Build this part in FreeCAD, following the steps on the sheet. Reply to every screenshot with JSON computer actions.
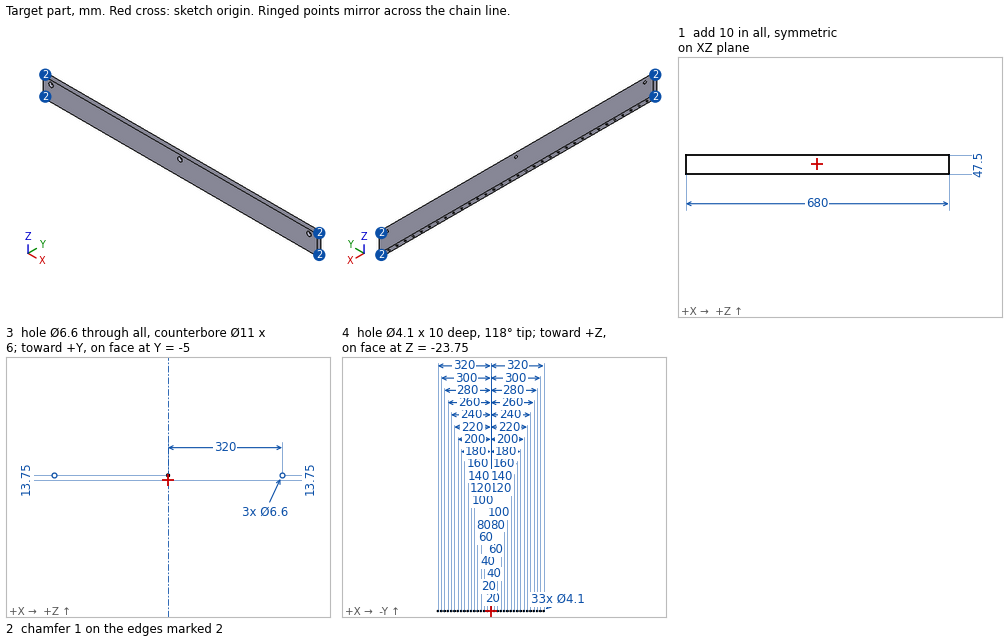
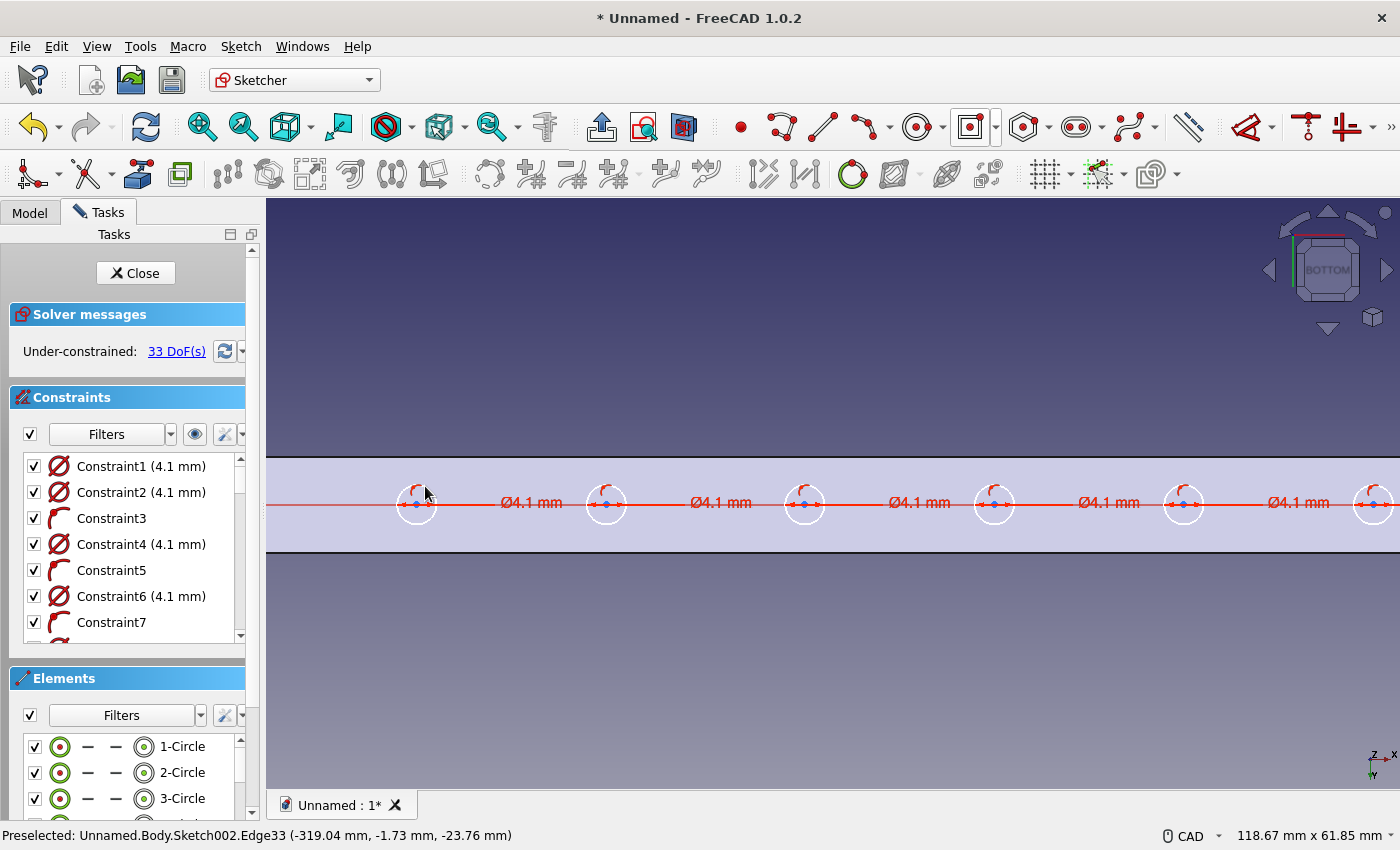
{"action": "scroll", "coordinate": [427, 492], "scroll_direction": "down", "scroll_amount": 11}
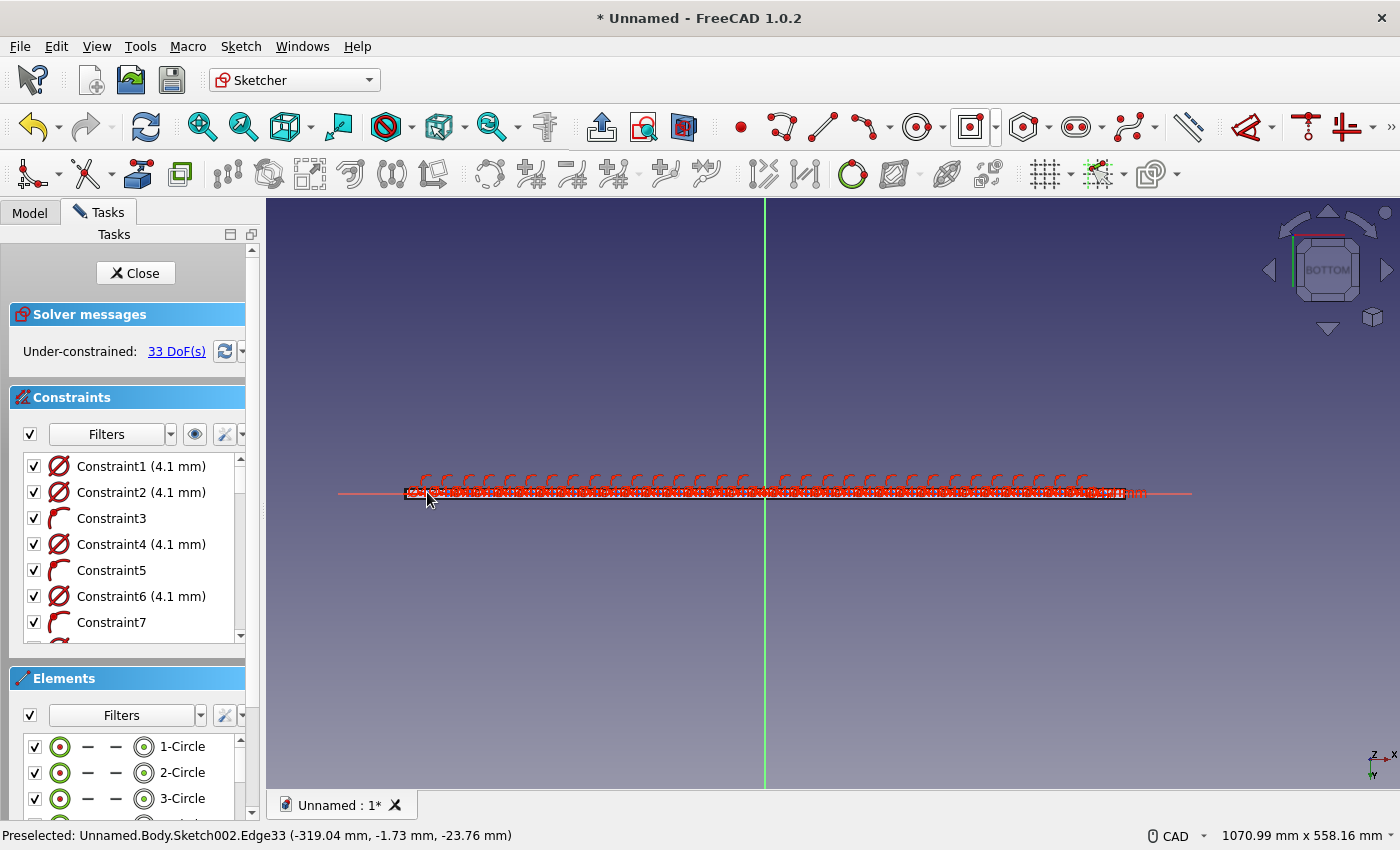
{"action": "left_click", "coordinate": [1104, 495]}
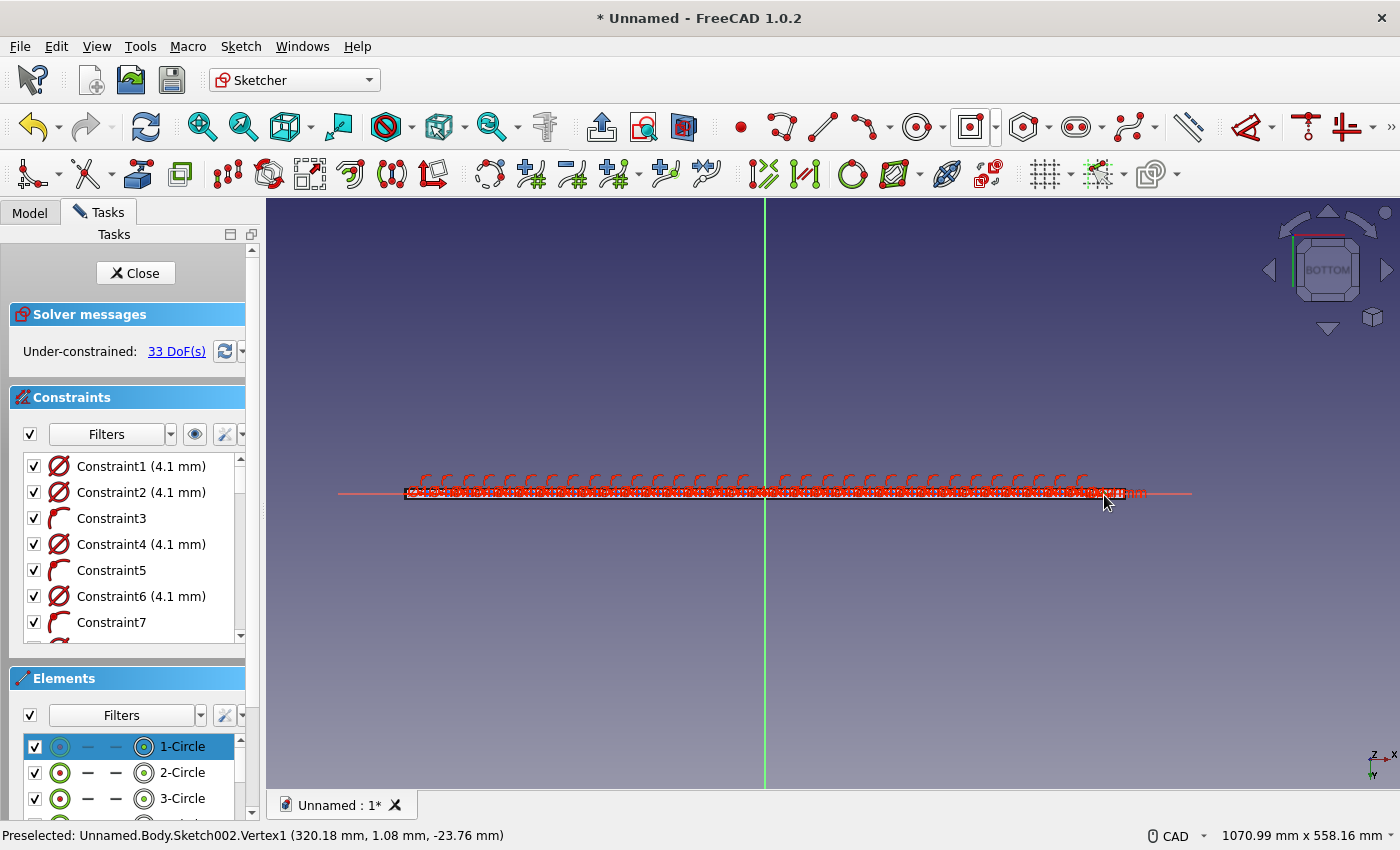
{"action": "left_click", "coordinate": [361, 494]}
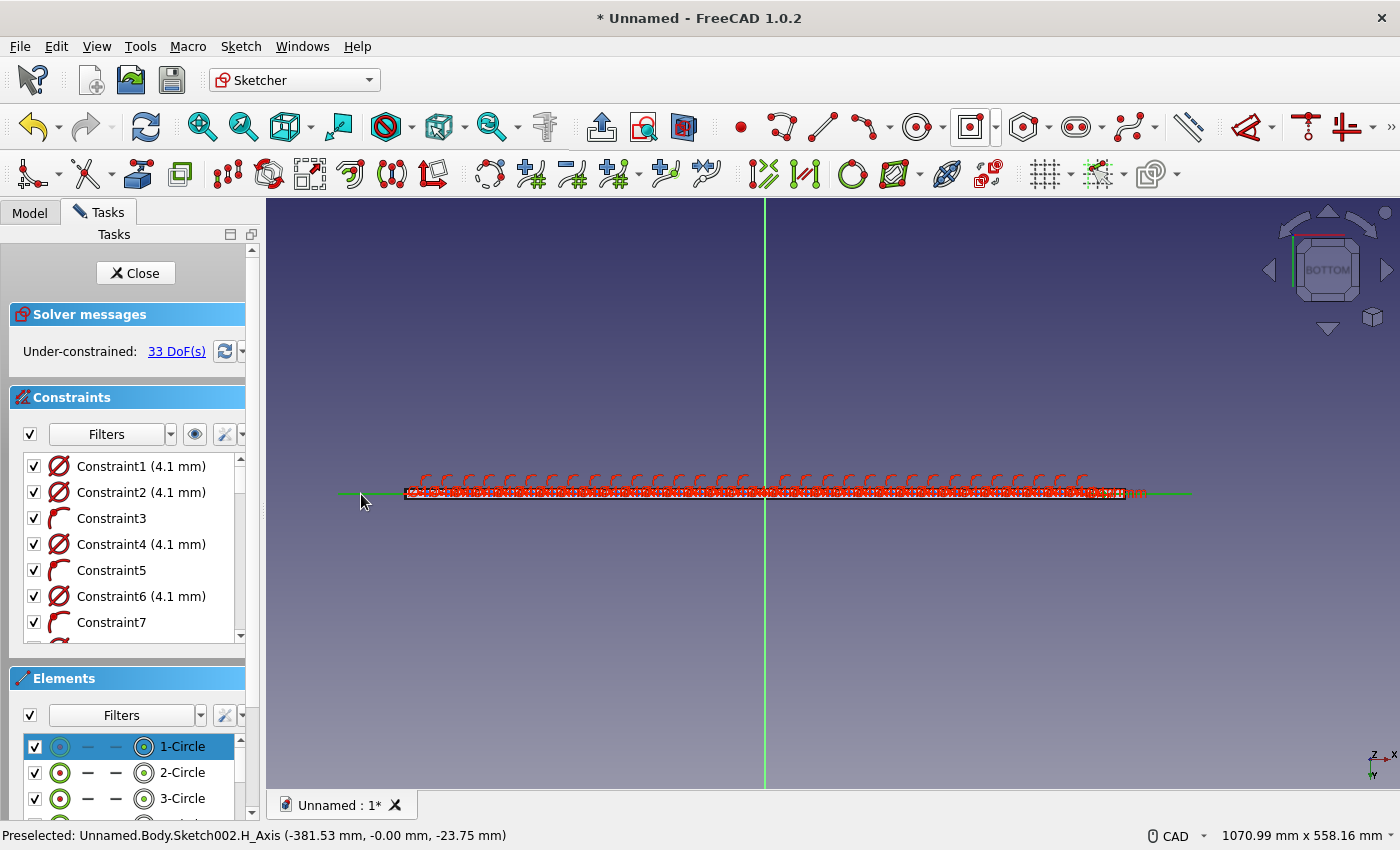
{"action": "left_click", "coordinate": [1306, 128]}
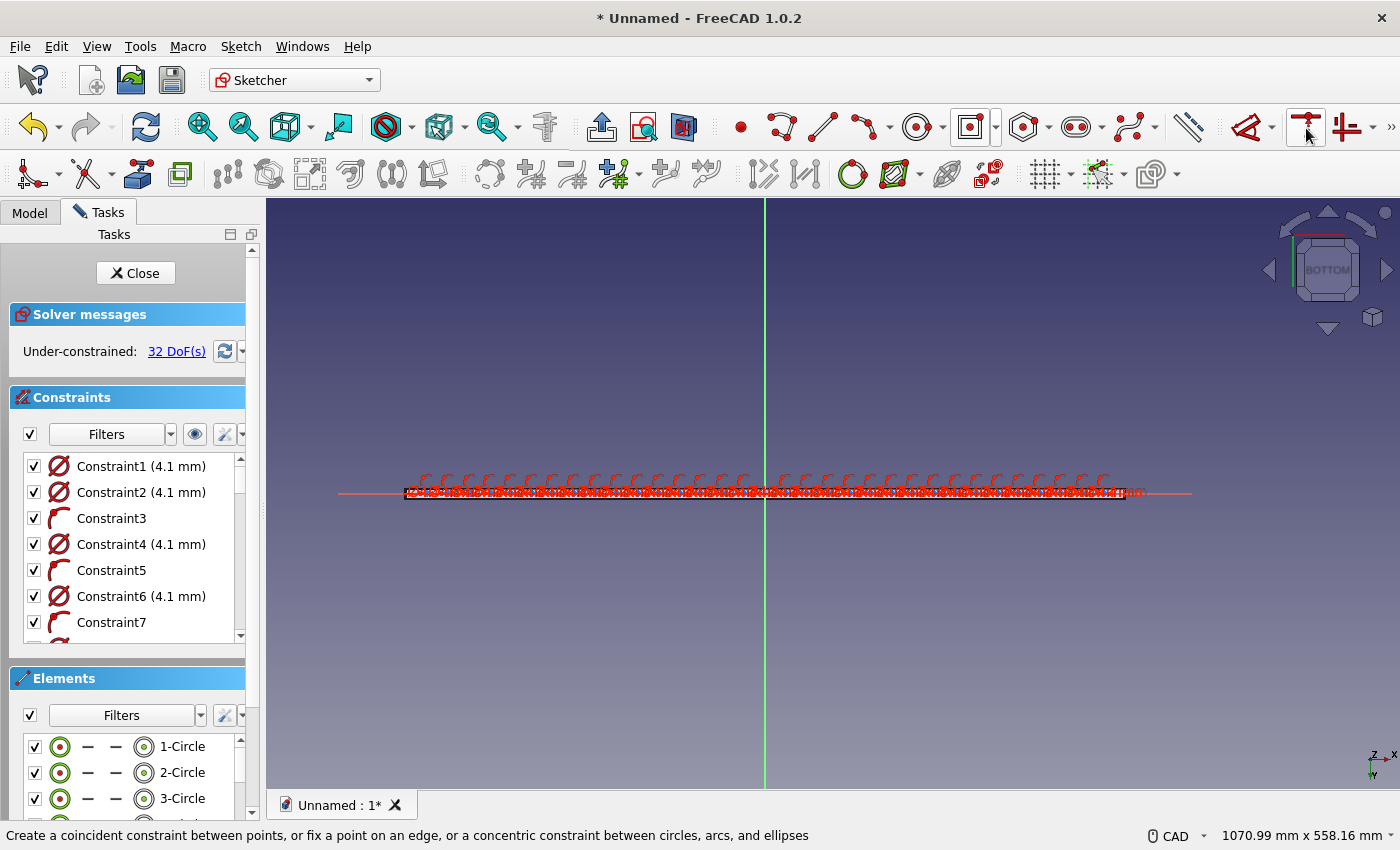
{"action": "left_click", "coordinate": [1246, 128]}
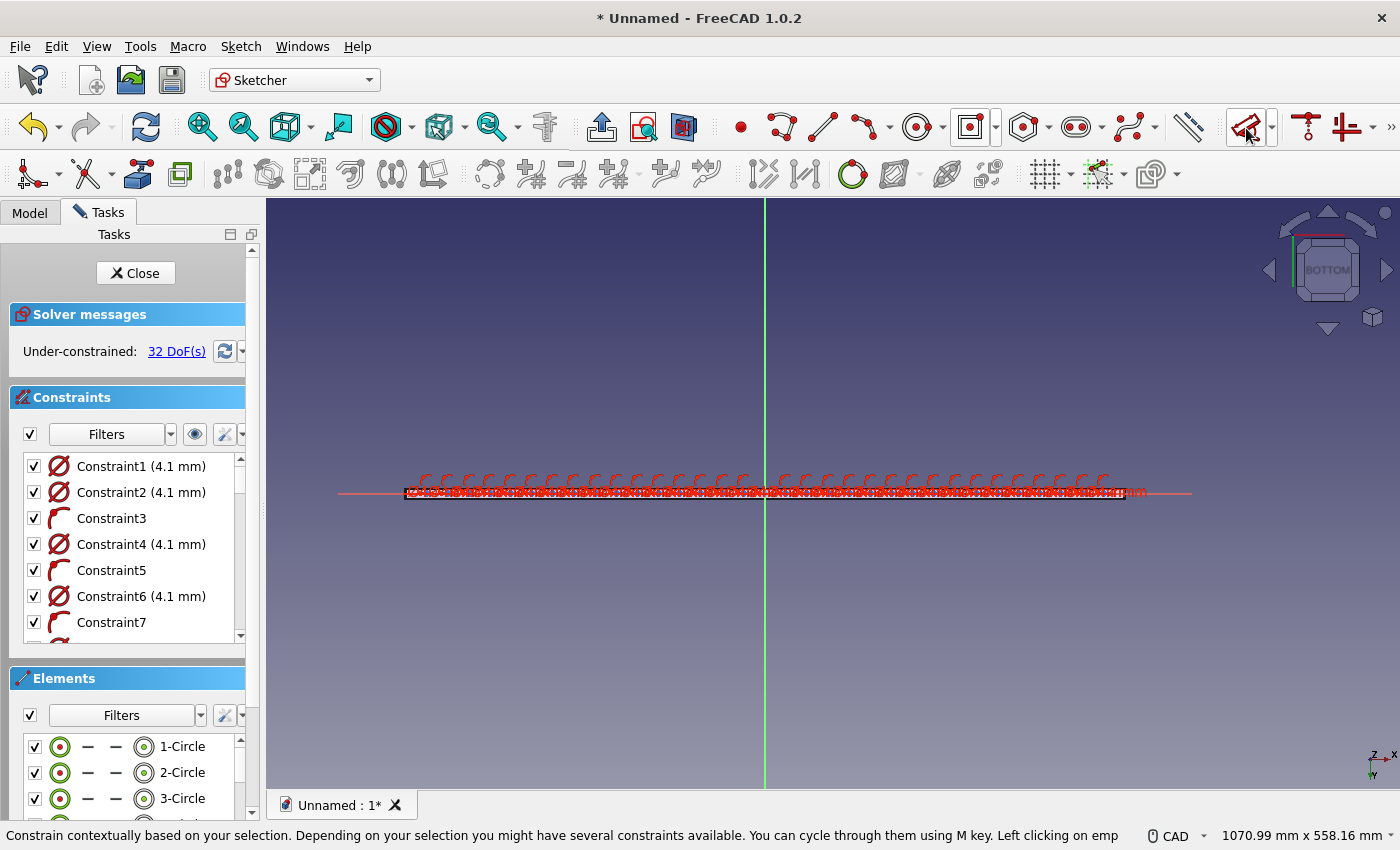
{"action": "left_click", "coordinate": [850, 494]}
{"action": "left_click", "coordinate": [807, 528]}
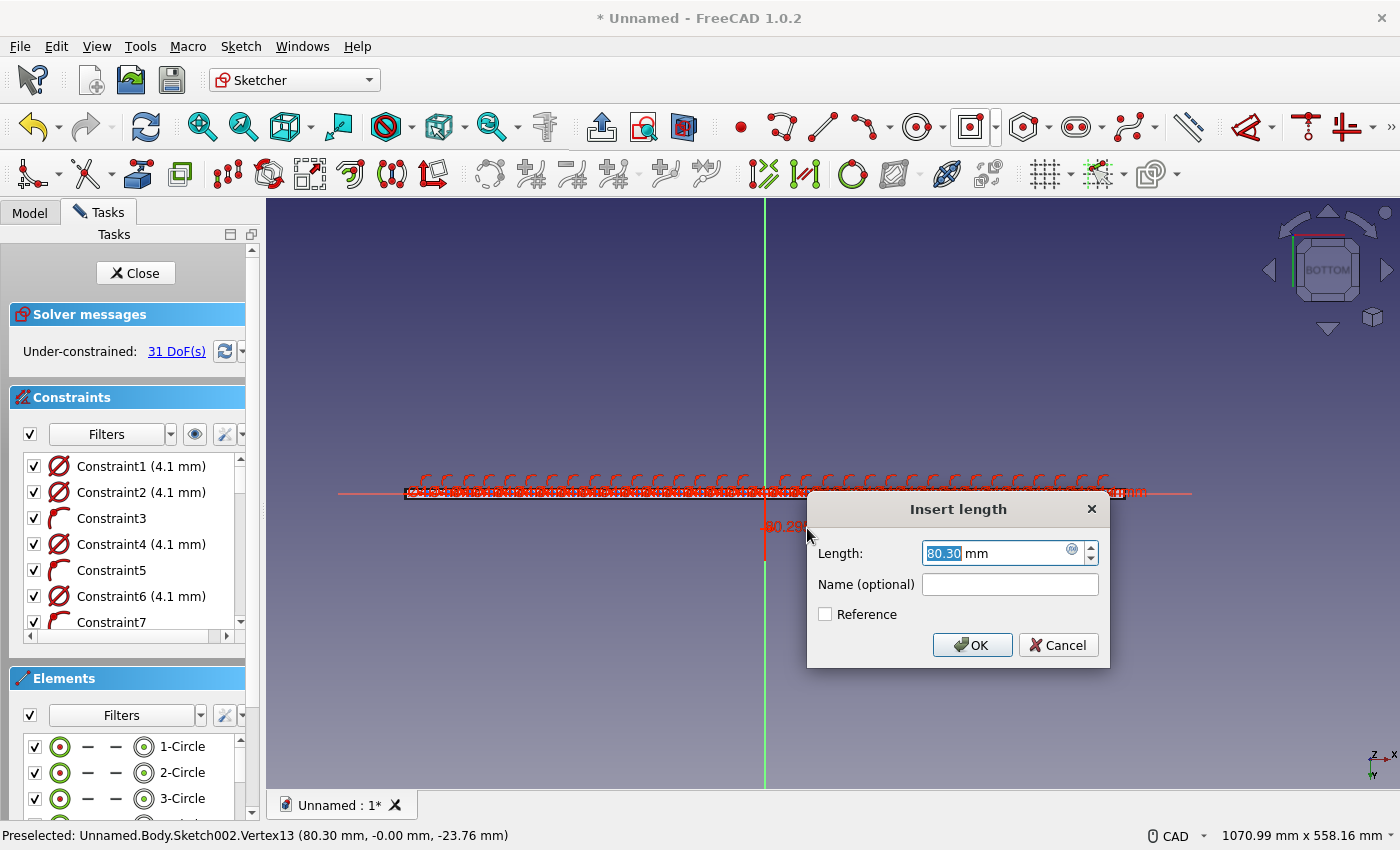
{"action": "type", "text": "80"}
{"action": "key", "text": "Return"}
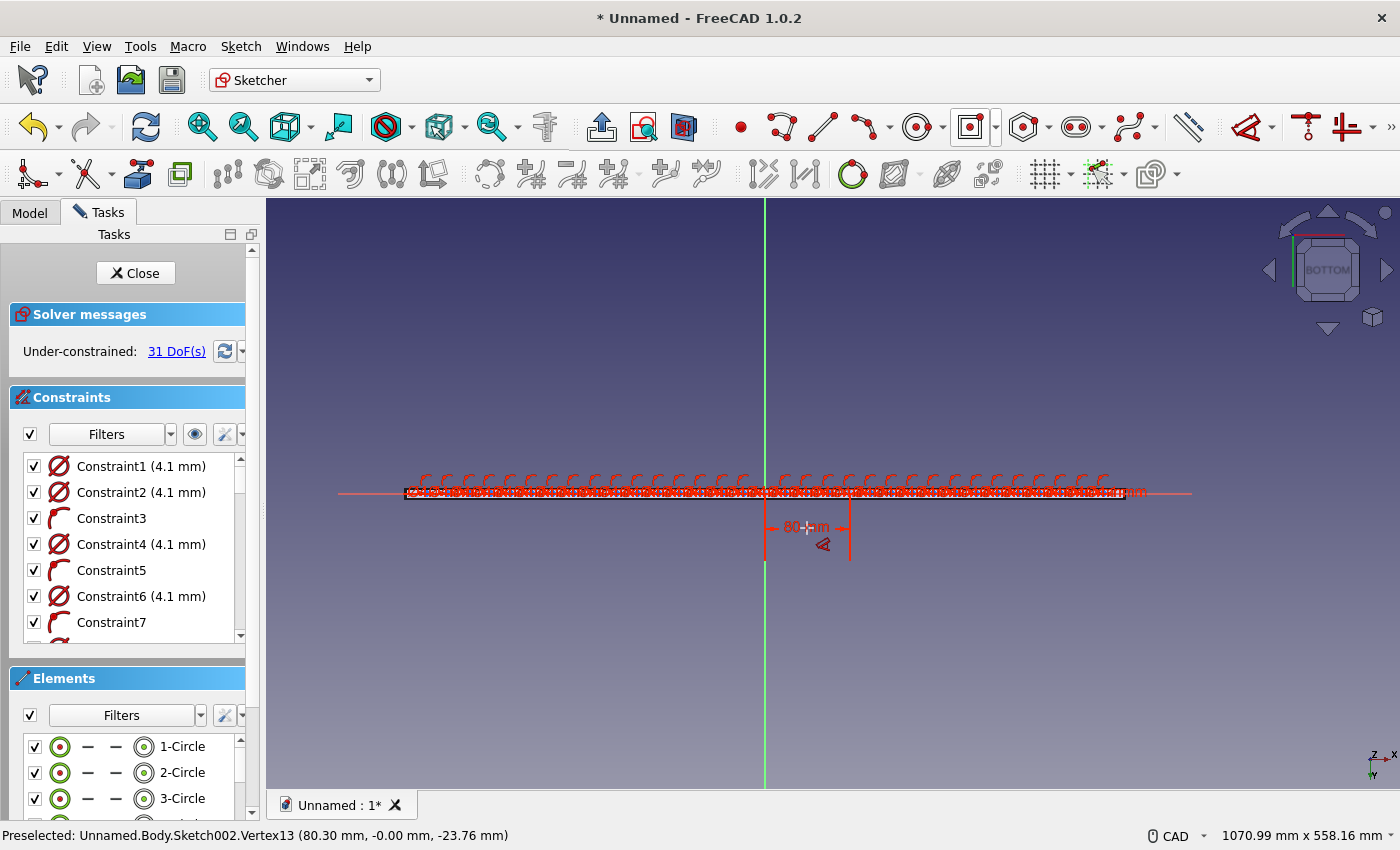
{"action": "left_click", "coordinate": [829, 494]}
{"action": "left_click", "coordinate": [797, 460]}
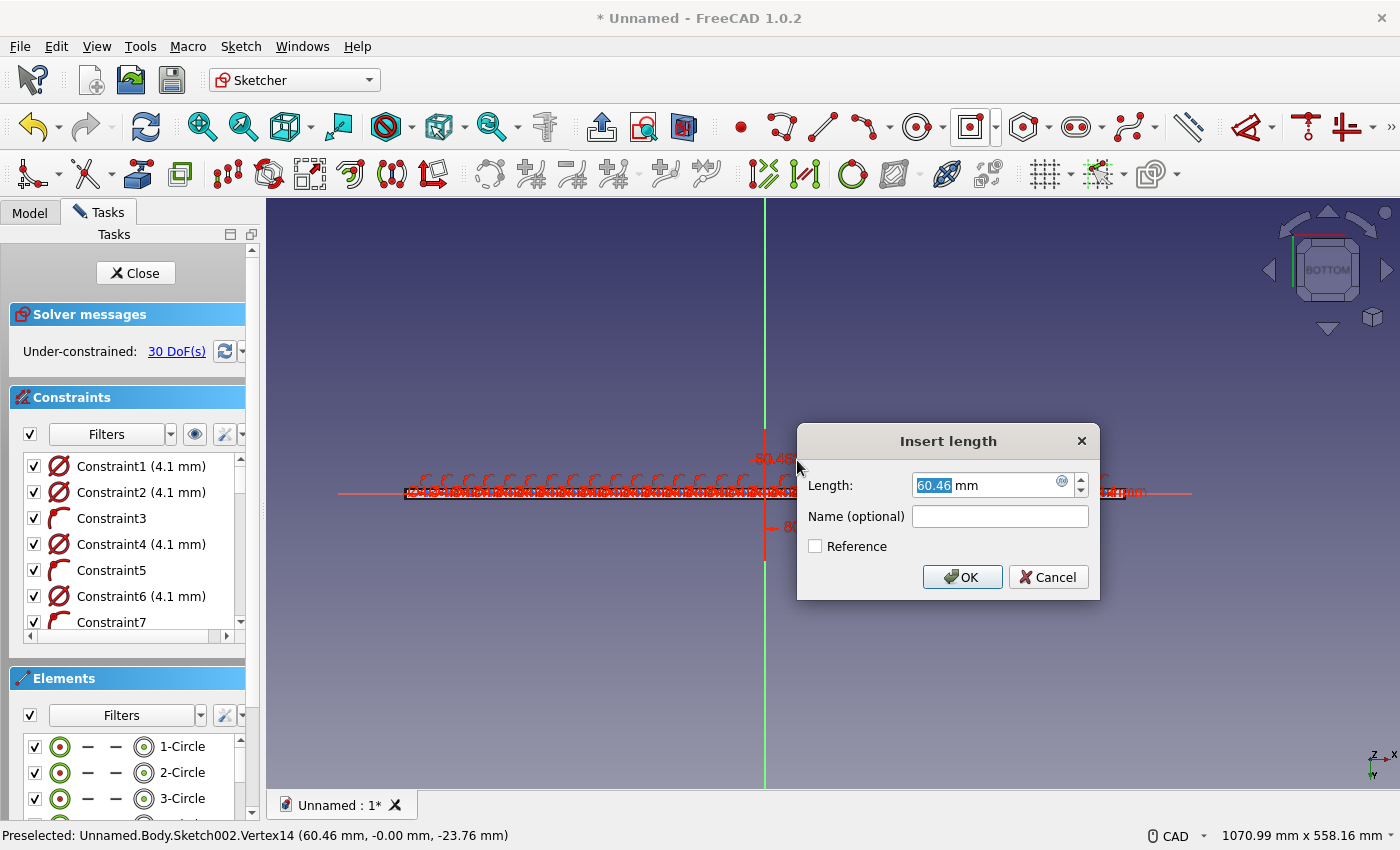
{"action": "type", "text": "60"}
{"action": "key", "text": "Return"}